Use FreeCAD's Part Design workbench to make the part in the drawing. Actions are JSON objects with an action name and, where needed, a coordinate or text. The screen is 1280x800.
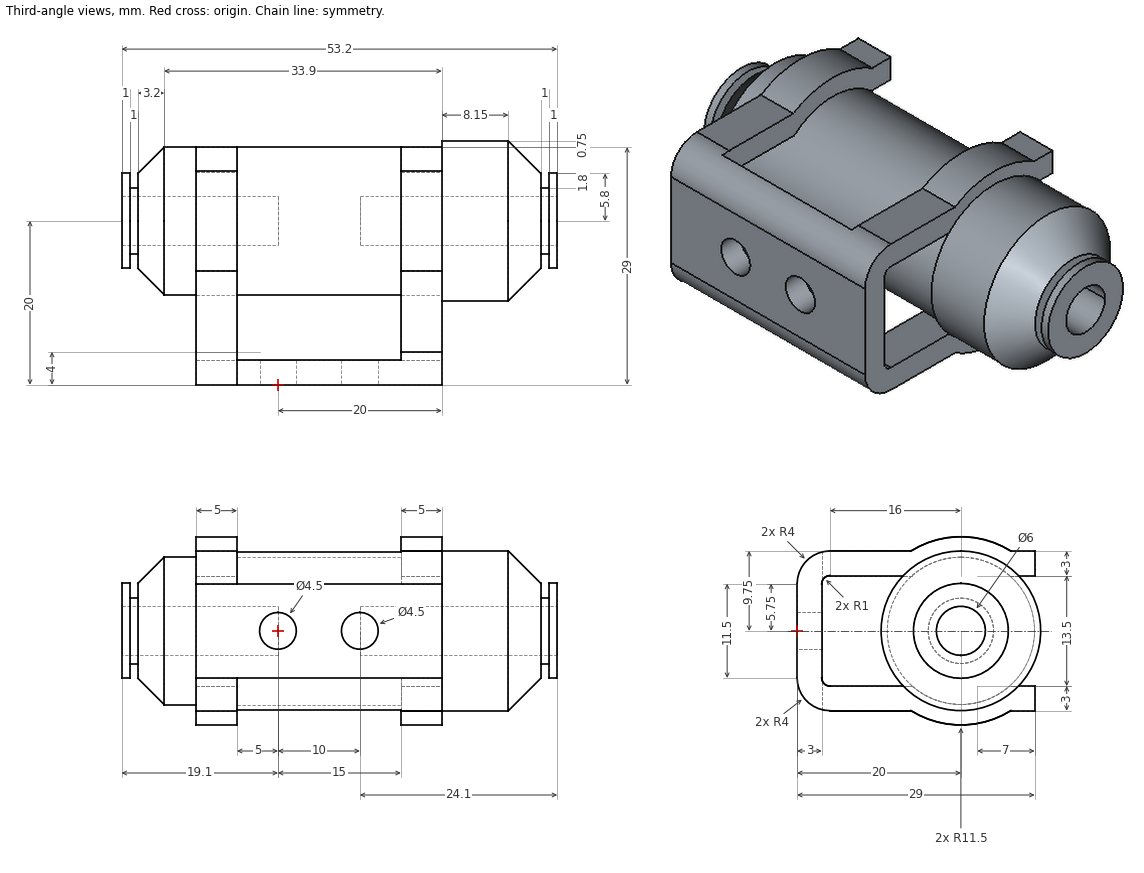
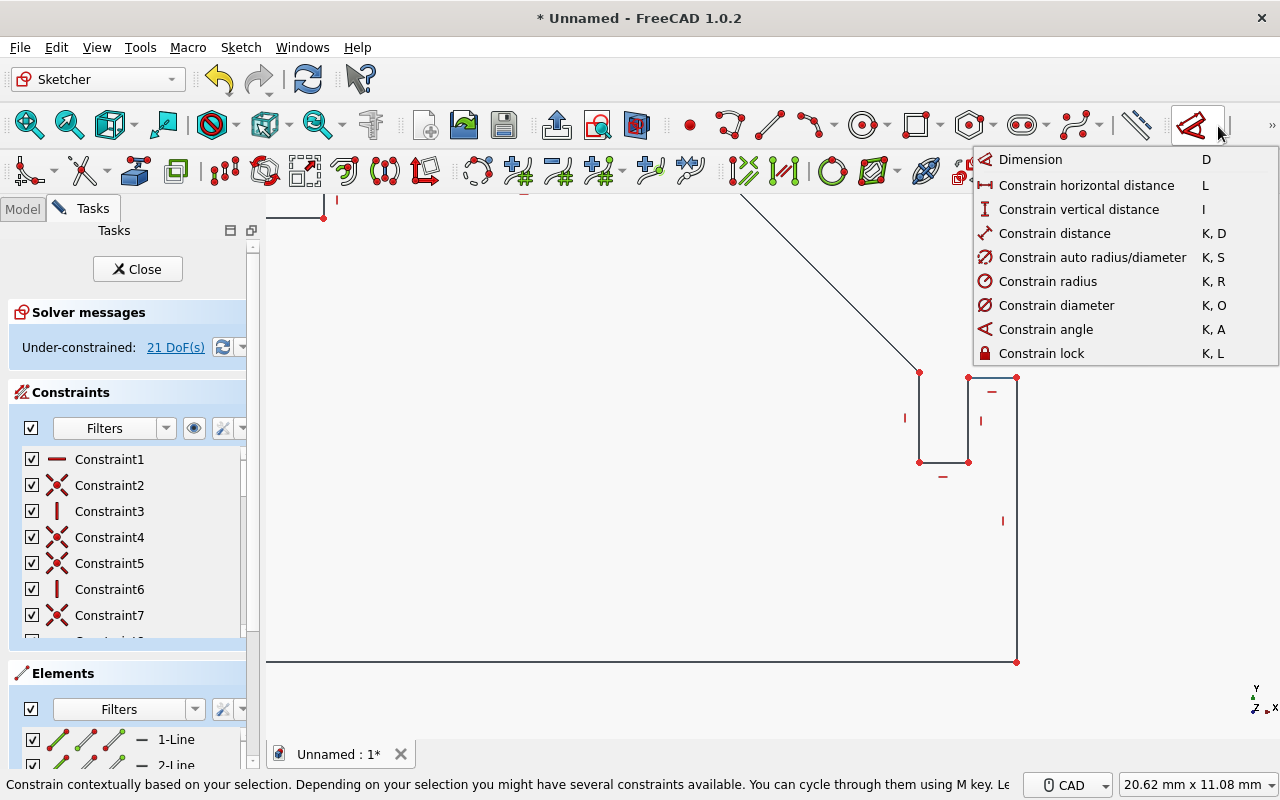
{"action": "left_click", "coordinate": [1126, 185]}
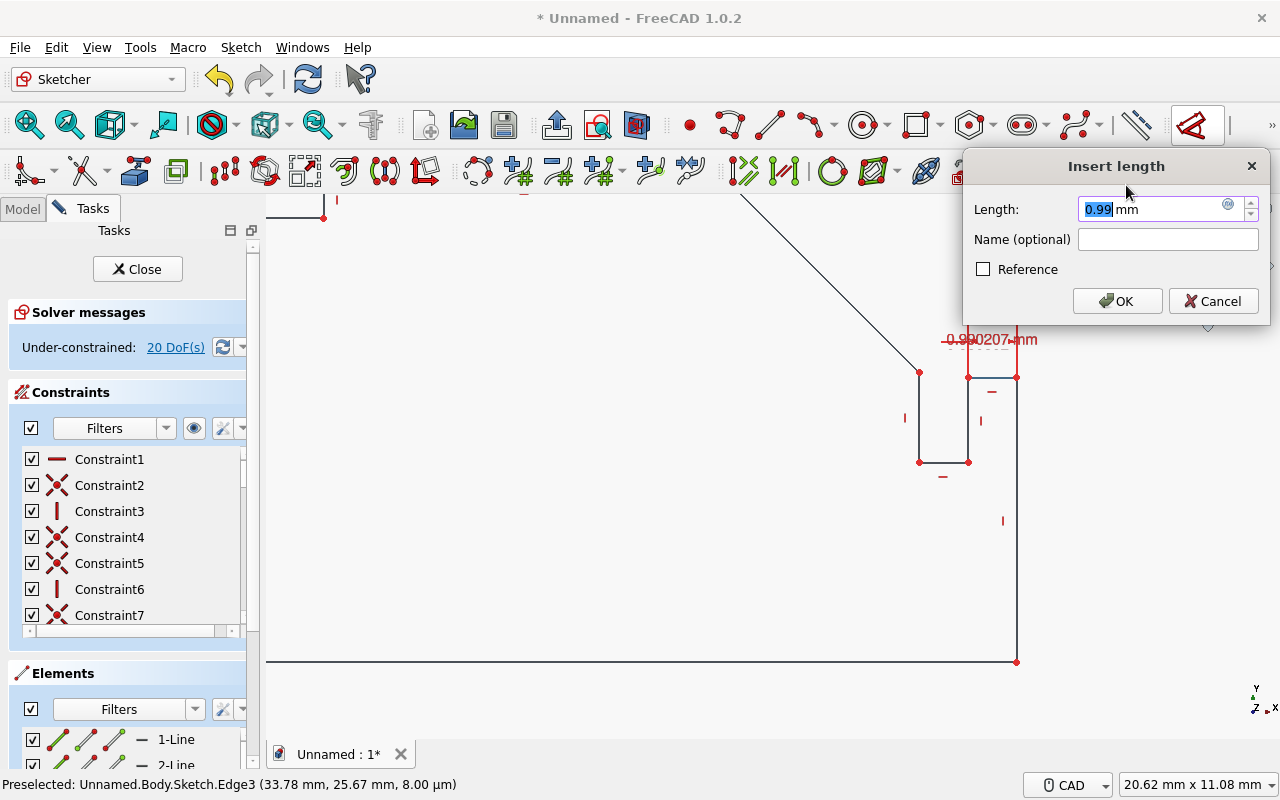
{"action": "type", "text": "1"}
{"action": "key", "text": "Return"}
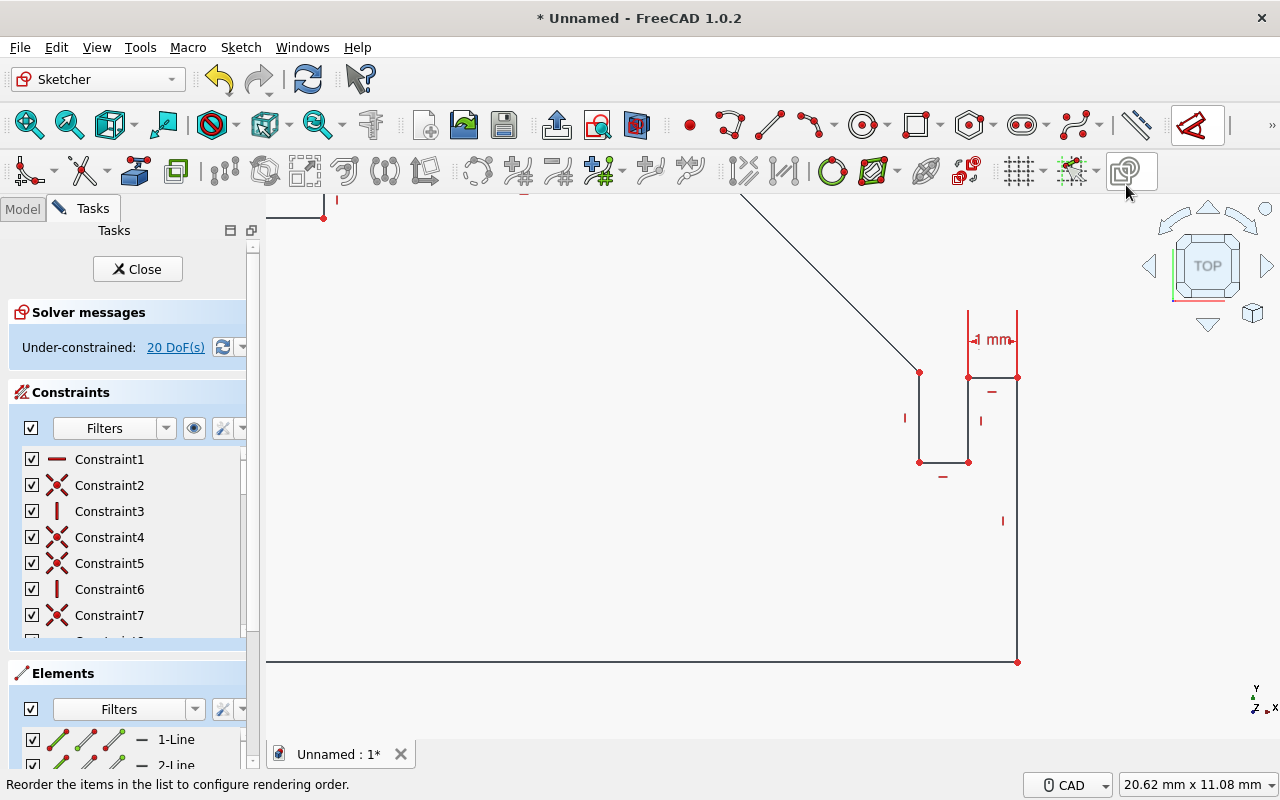
{"action": "left_click", "coordinate": [953, 463]}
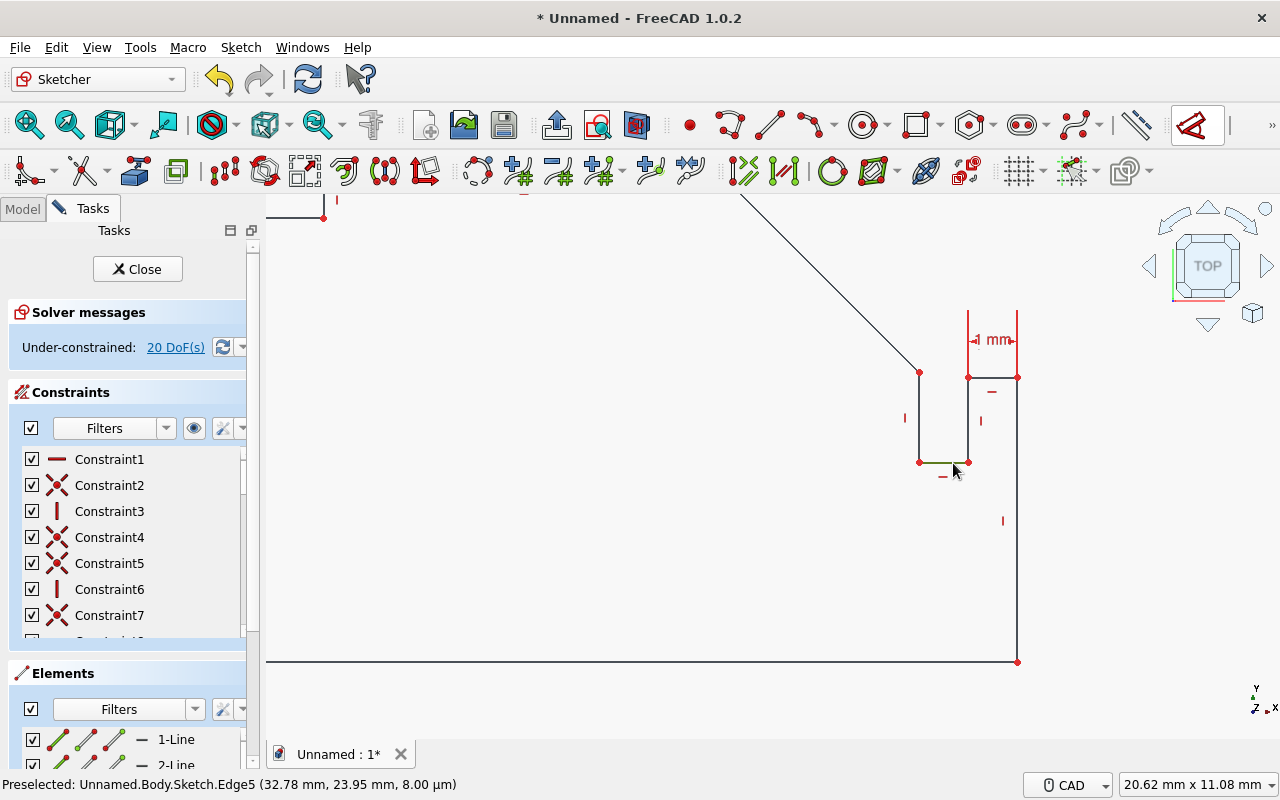
{"action": "left_click", "coordinate": [1218, 126]}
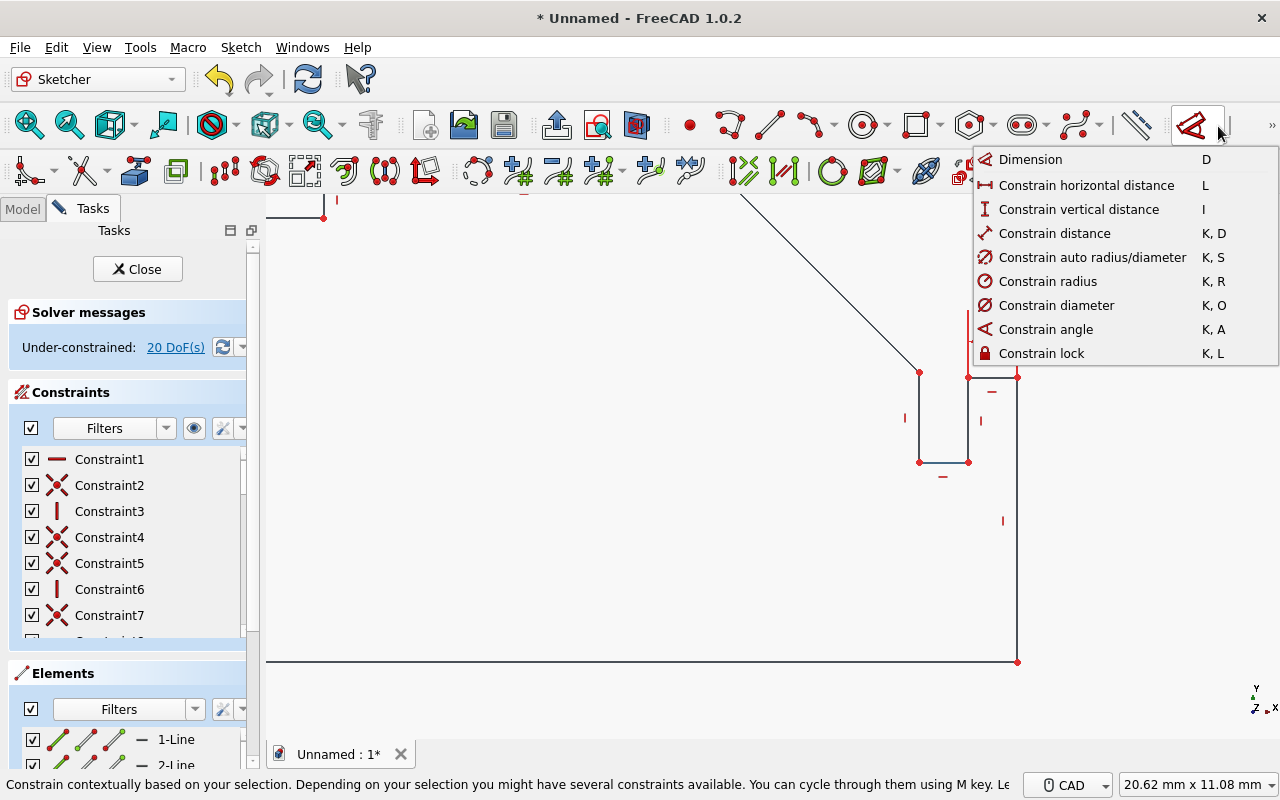
{"action": "left_click", "coordinate": [1126, 185]}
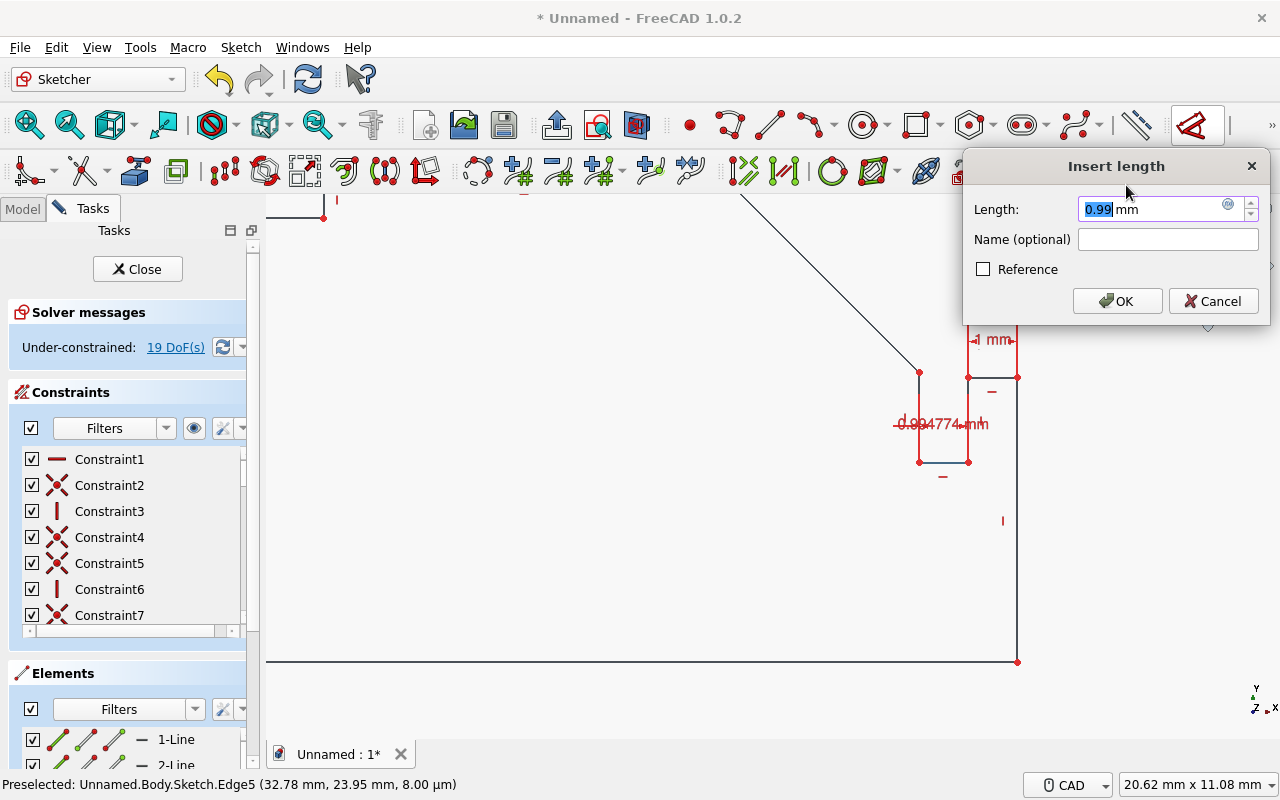
{"action": "type", "text": "1"}
{"action": "key", "text": "Return"}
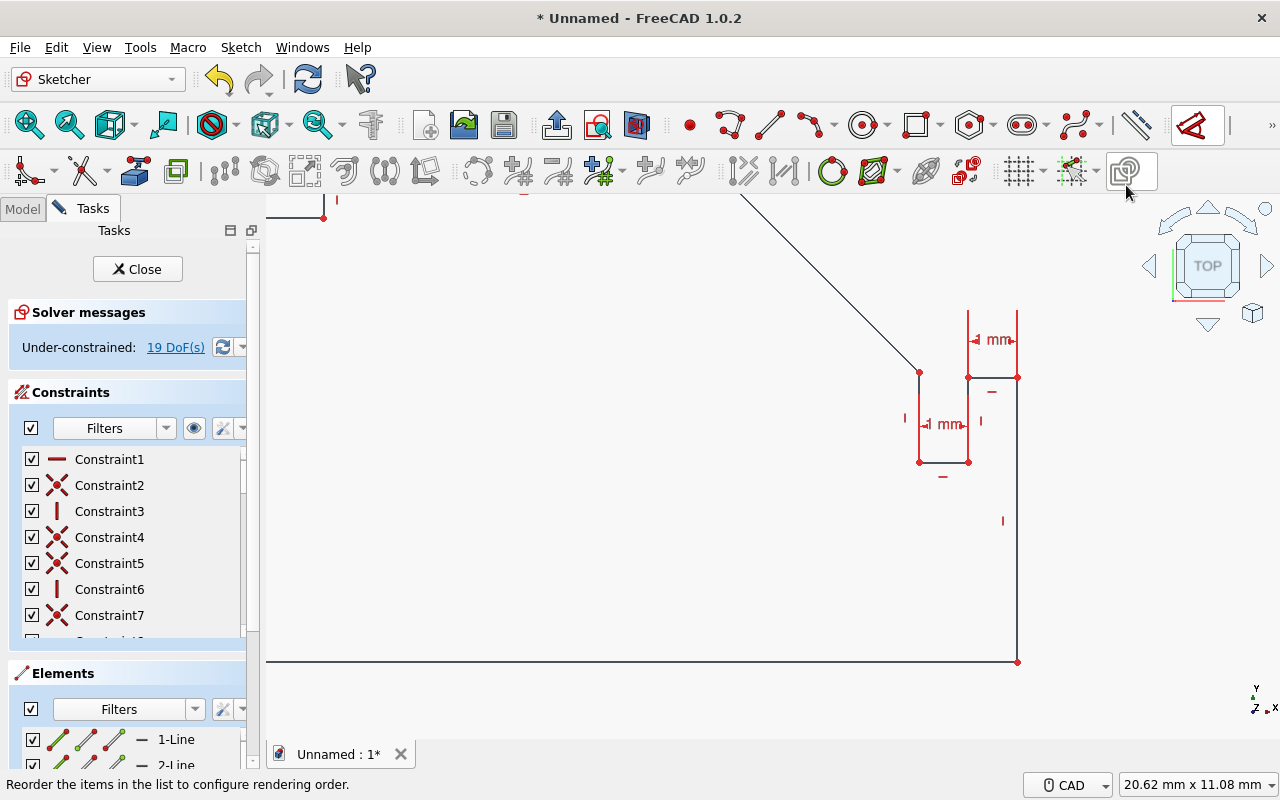
{"action": "scroll", "coordinate": [1005, 379], "scroll_direction": "down", "scroll_amount": 9}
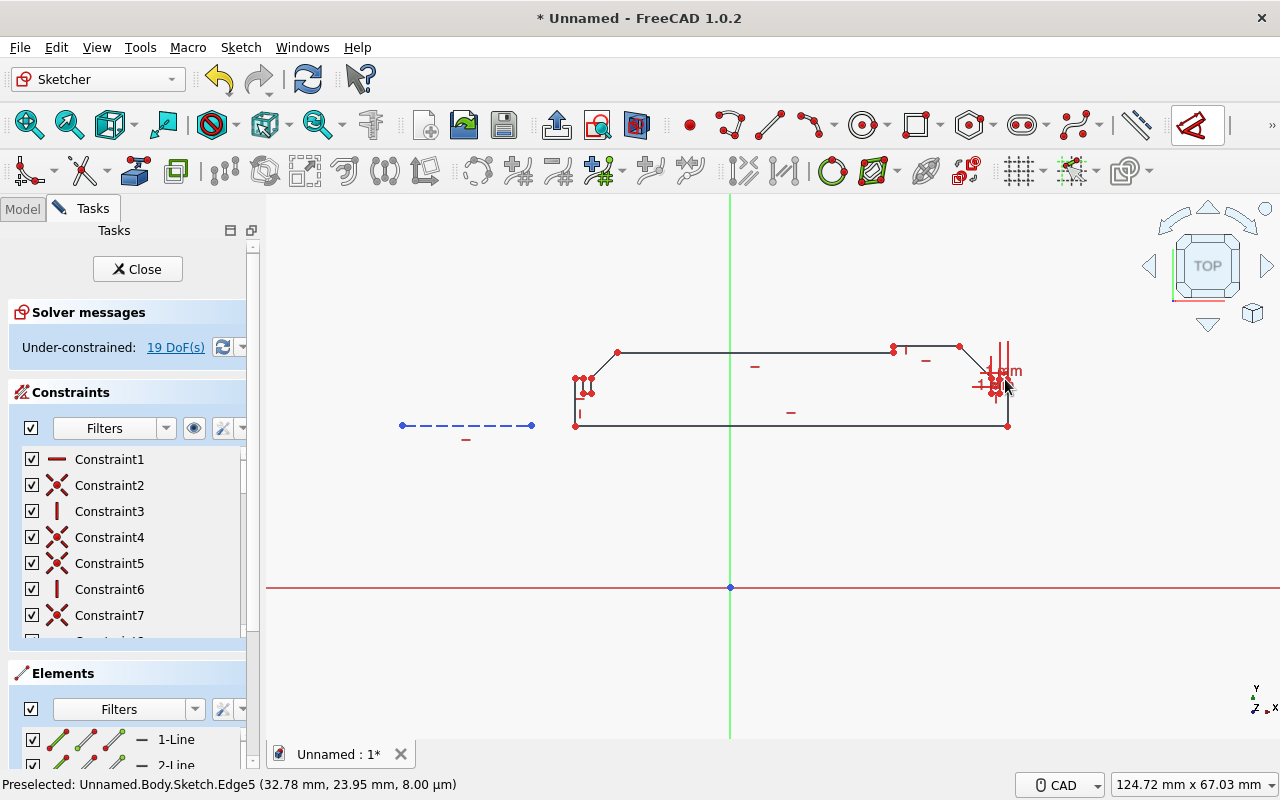
{"action": "scroll", "coordinate": [589, 394], "scroll_direction": "up", "scroll_amount": 9}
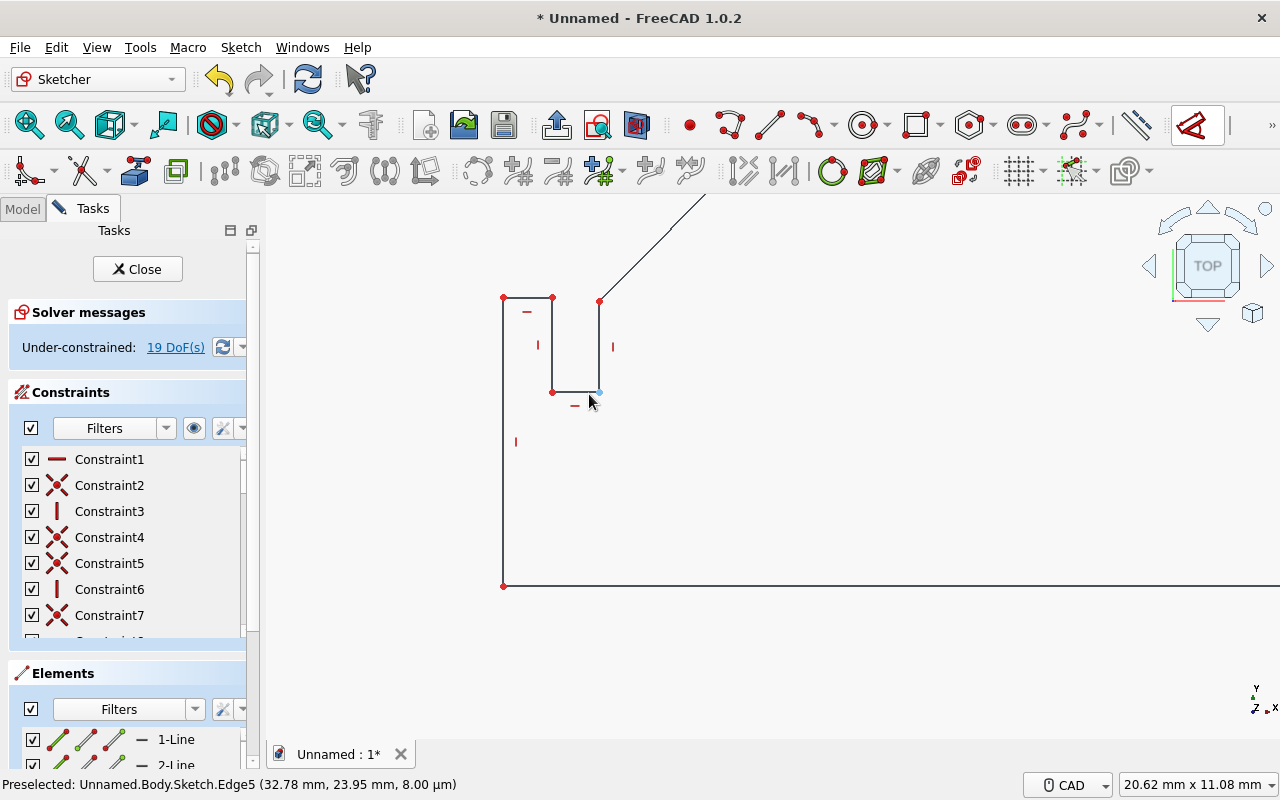
{"action": "left_click", "coordinate": [585, 392]}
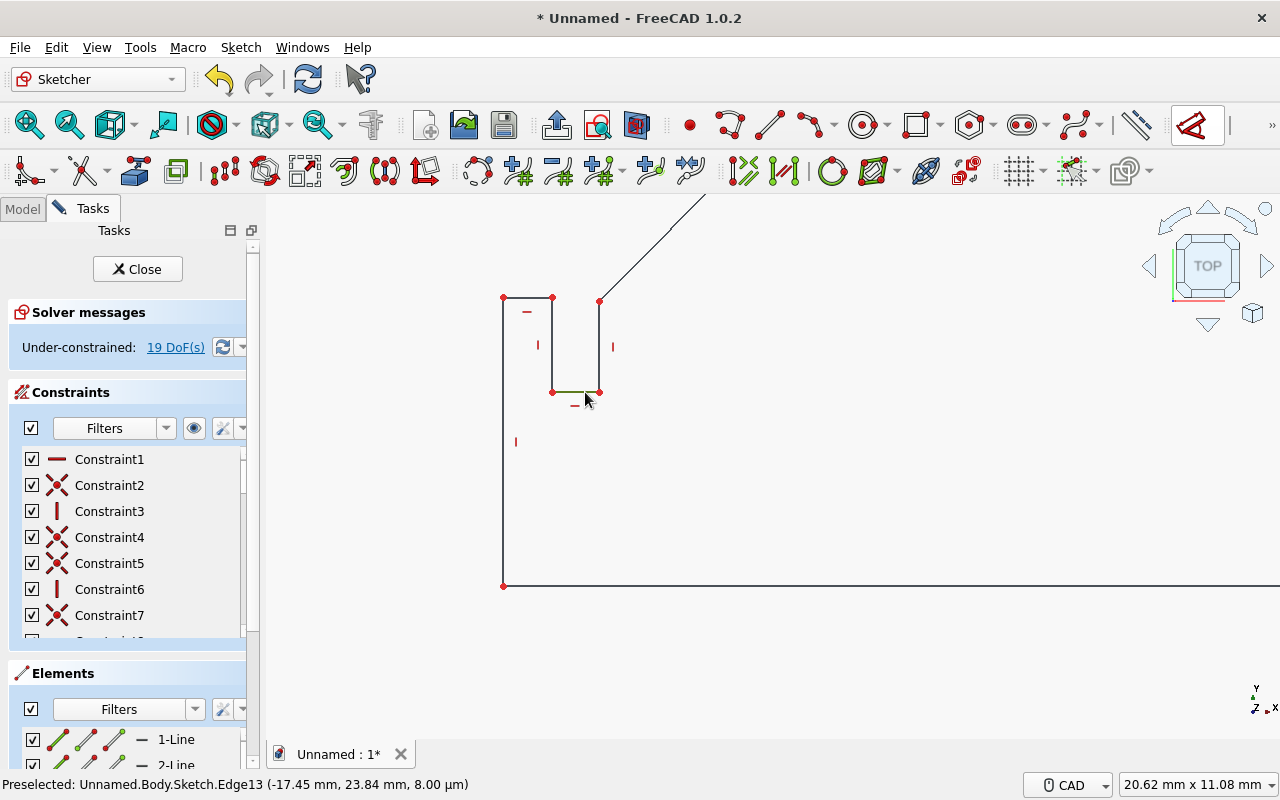
{"action": "left_click", "coordinate": [1218, 126]}